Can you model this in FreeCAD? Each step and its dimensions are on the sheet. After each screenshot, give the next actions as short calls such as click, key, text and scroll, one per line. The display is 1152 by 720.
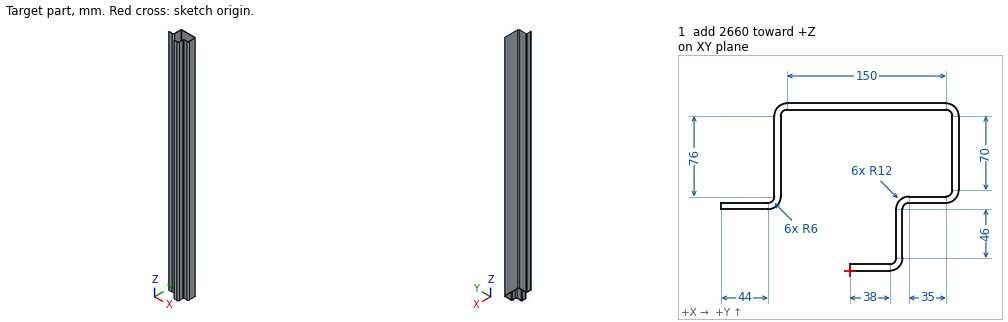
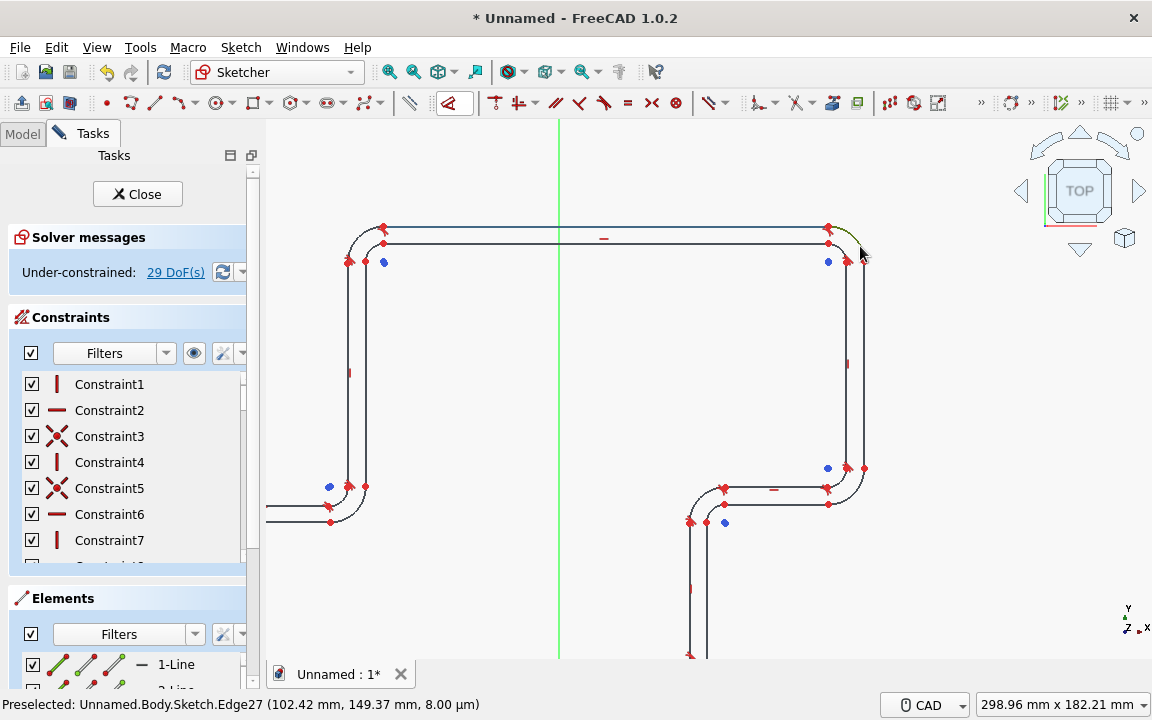
click(604, 104)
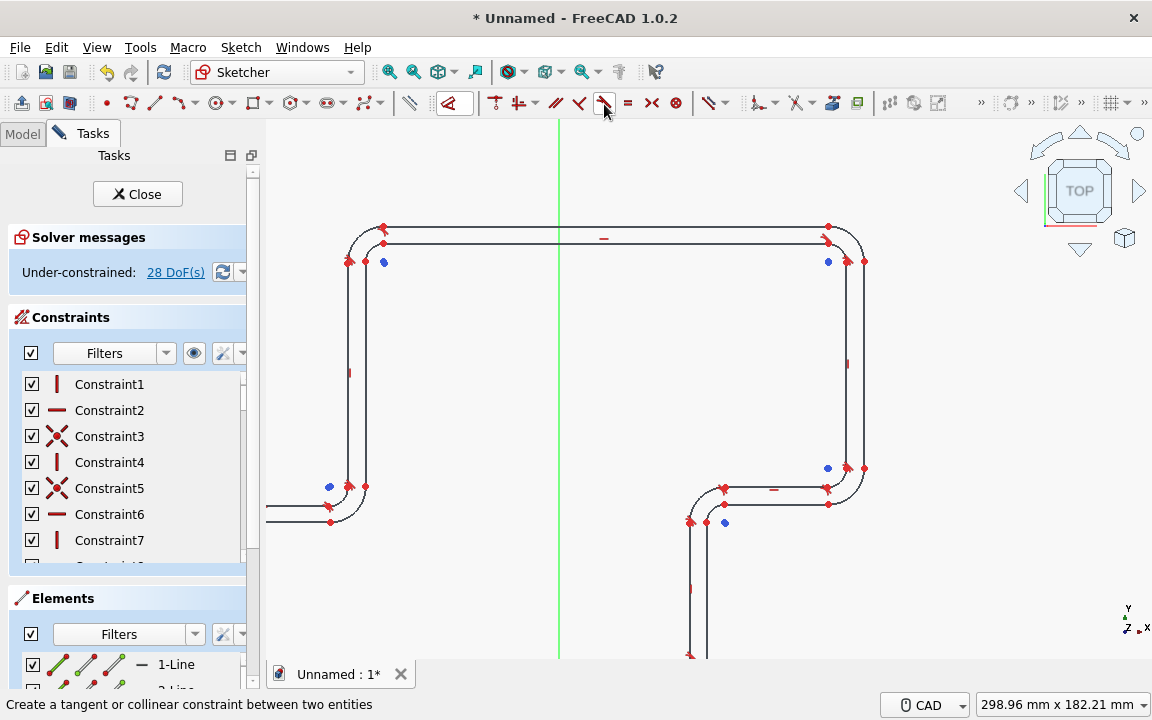
click(695, 227)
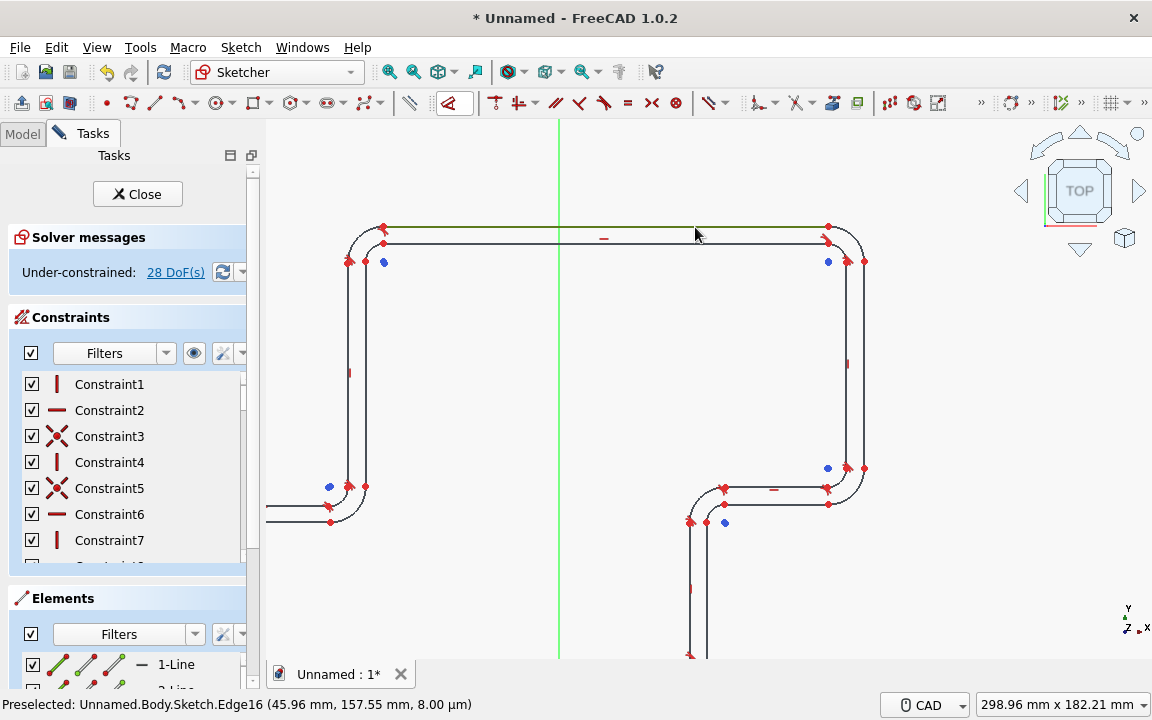
click(368, 231)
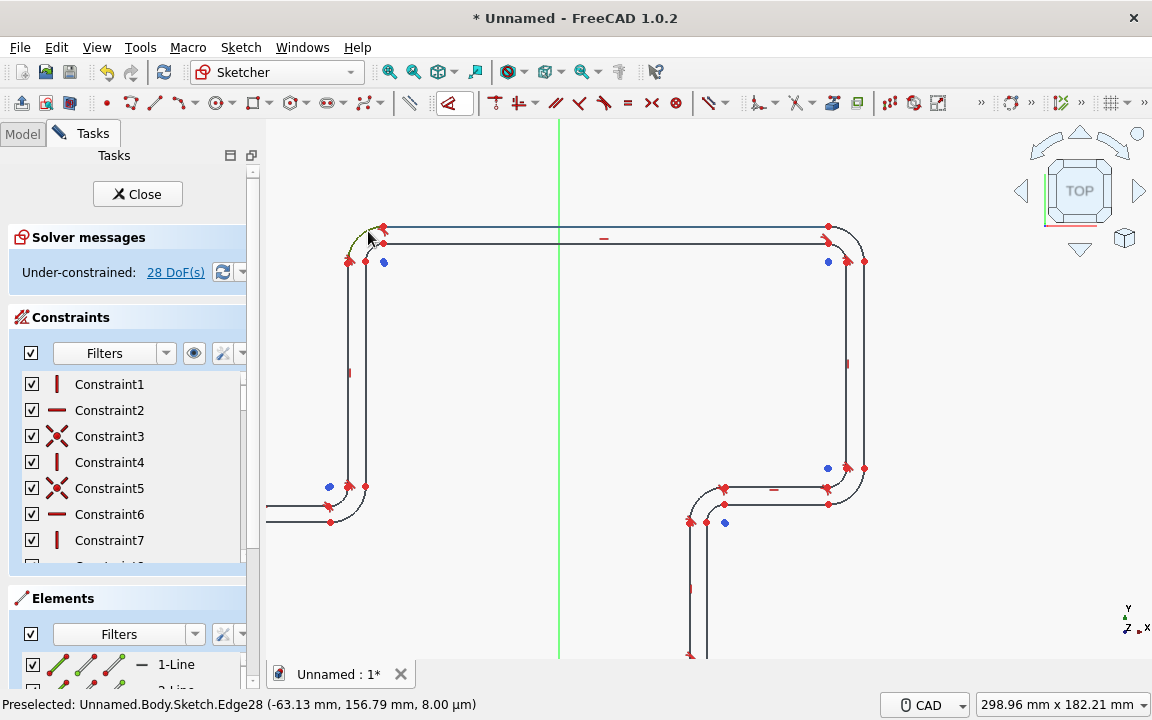
click(604, 104)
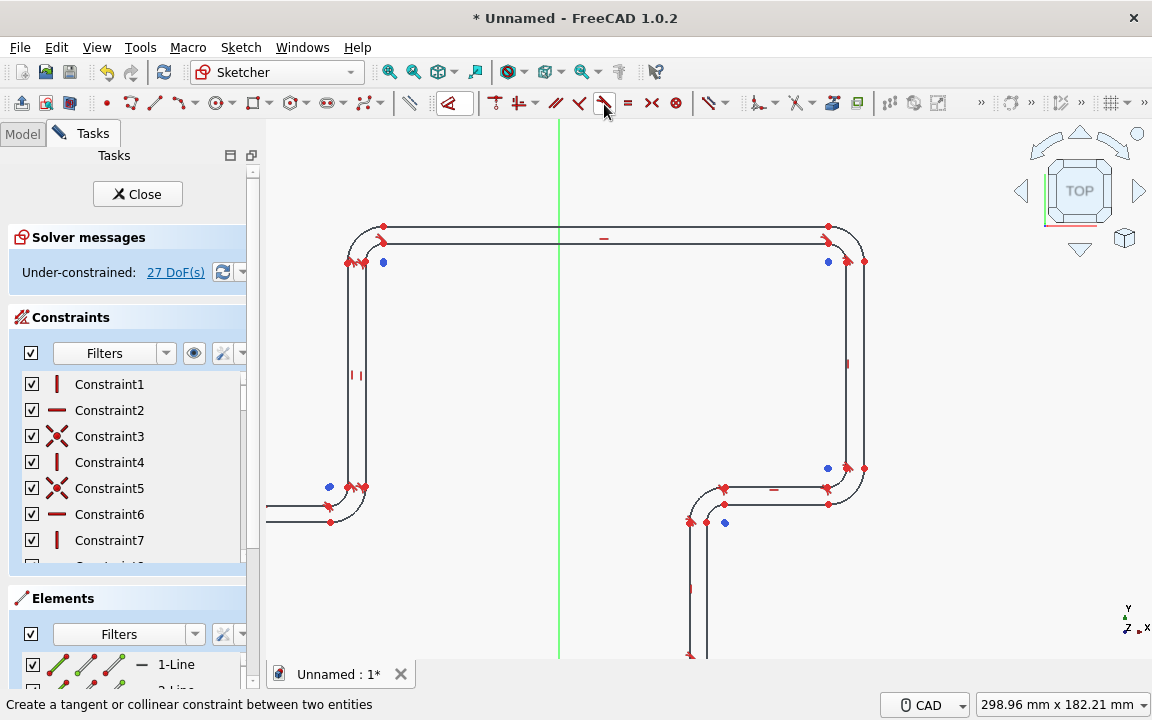
scroll(861, 246, down, 2)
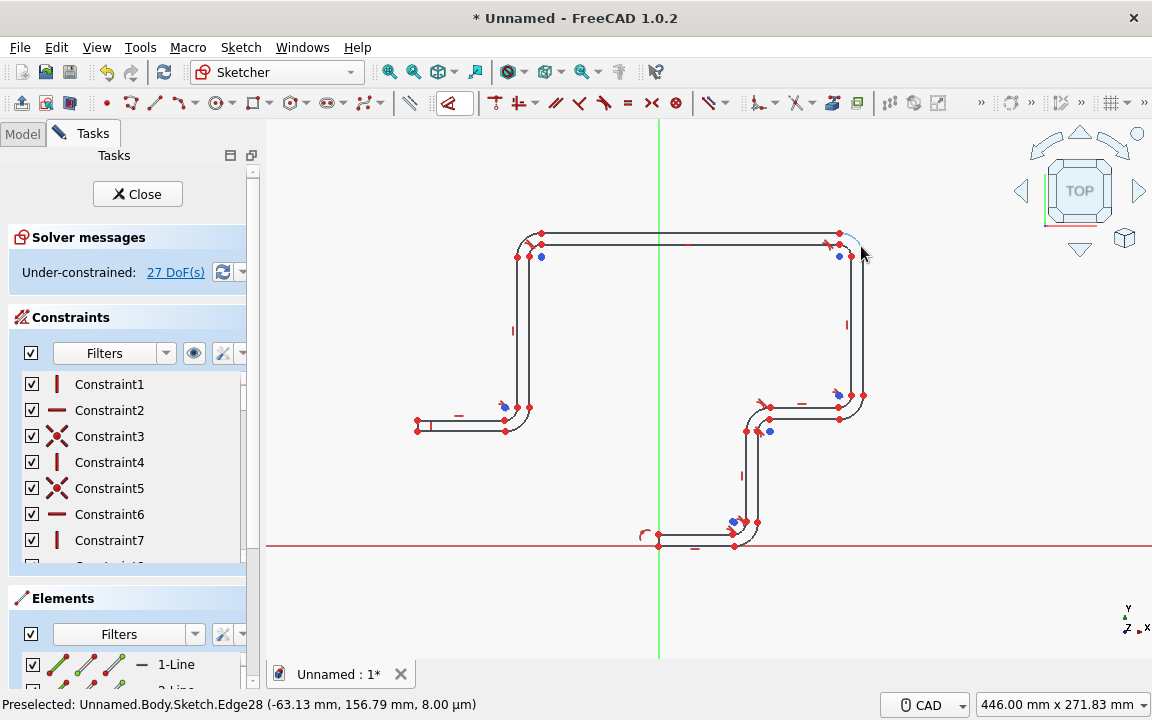
scroll(681, 546, up, 2)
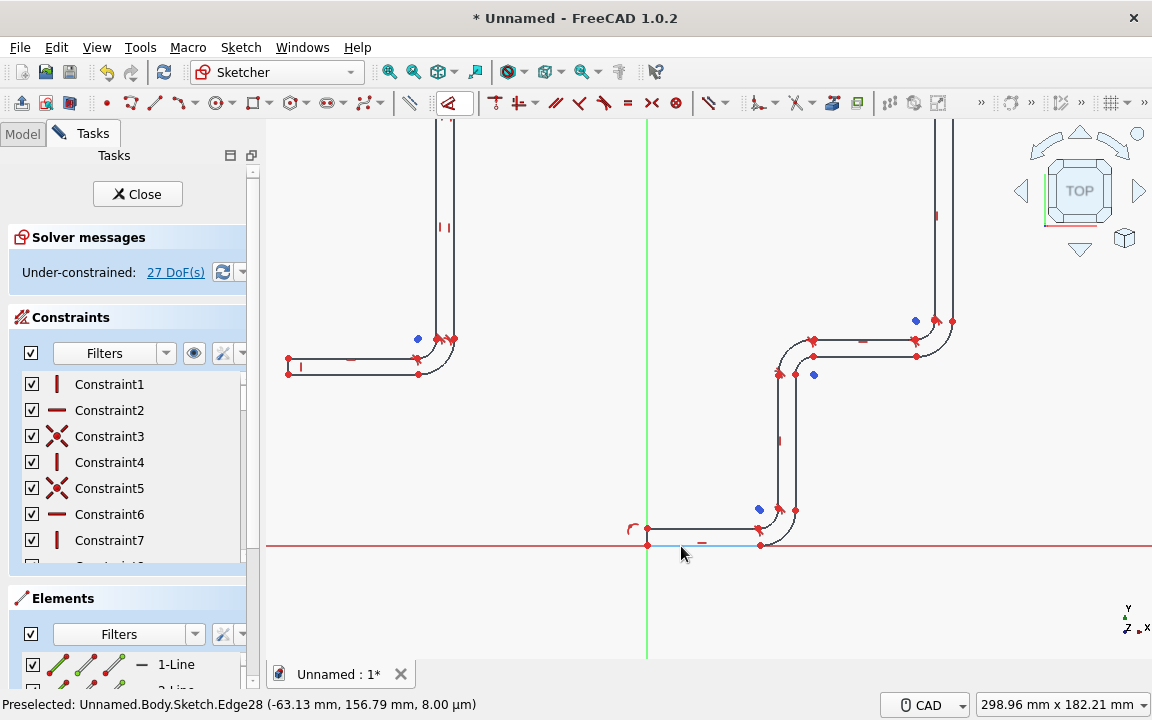
click(681, 546)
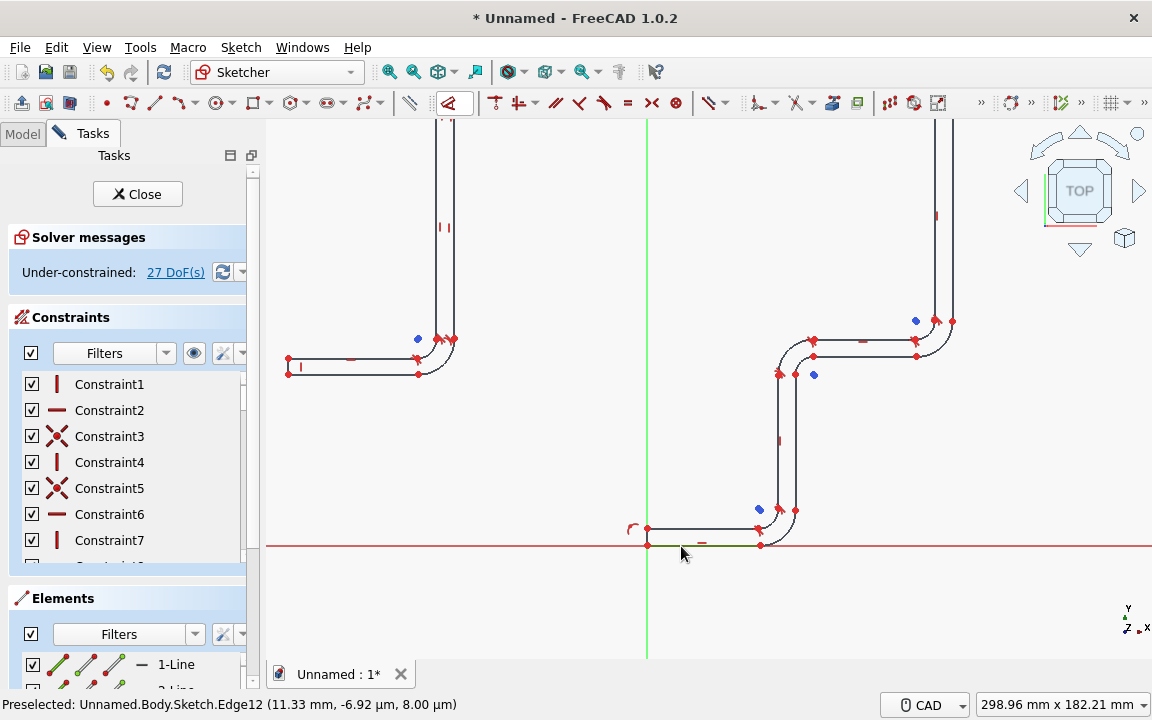
key(h)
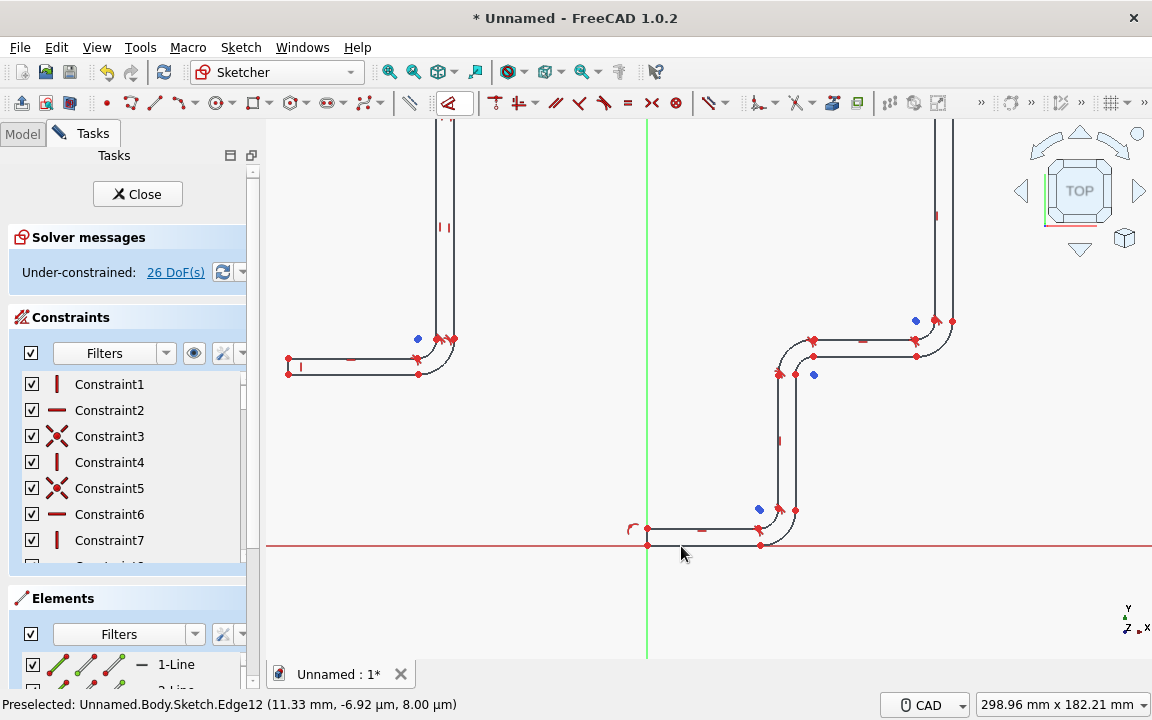
click(431, 353)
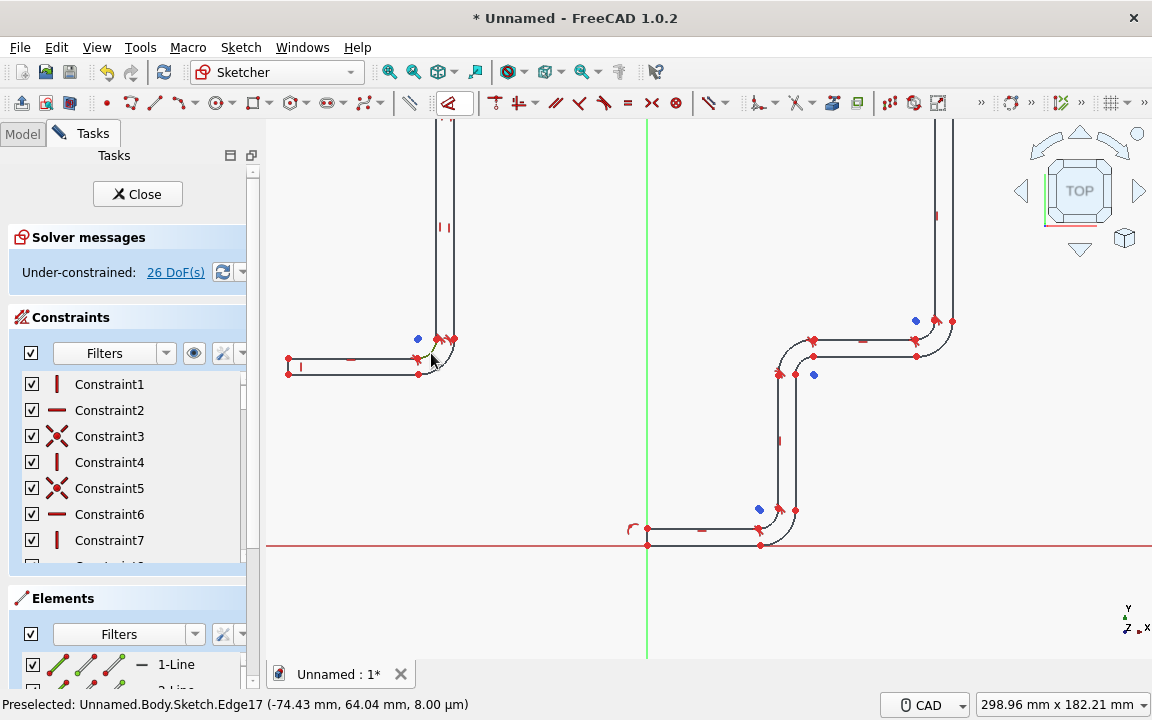
click(435, 371)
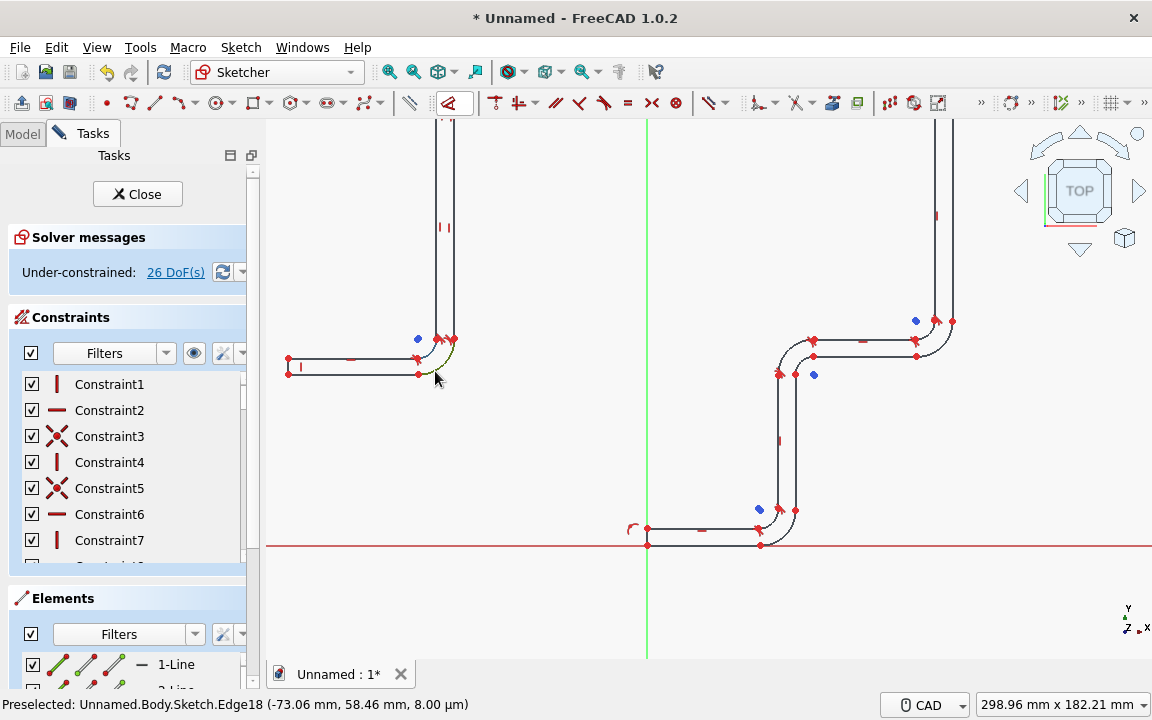
key(c)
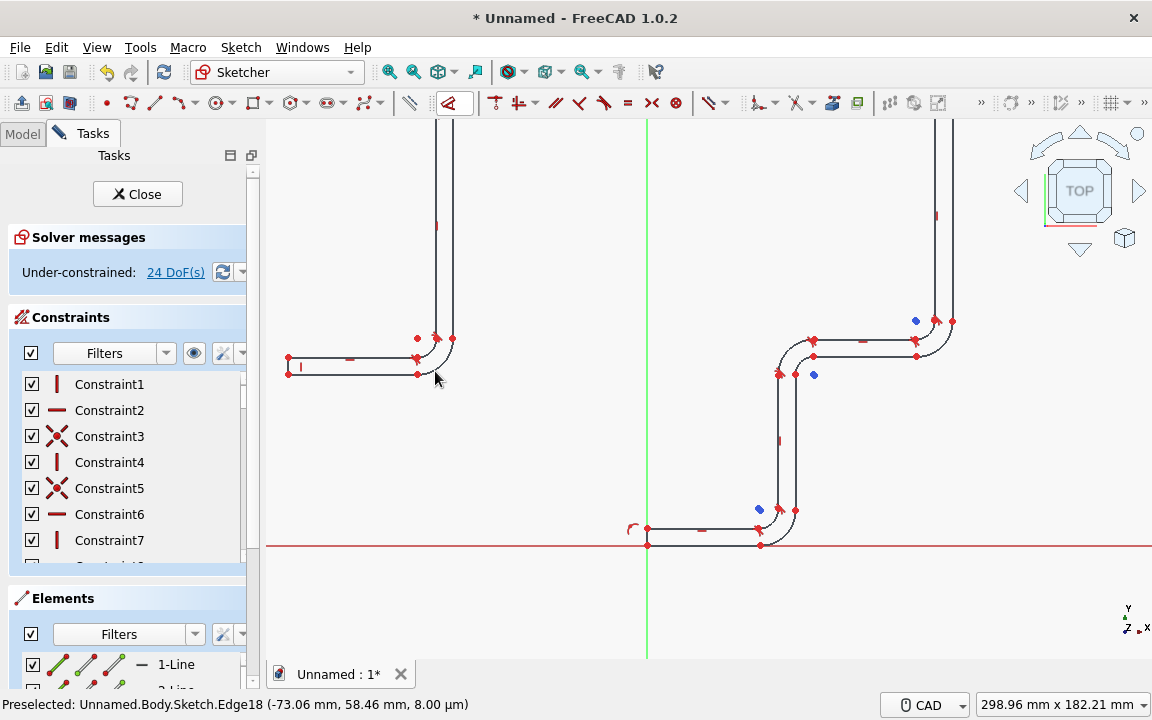
scroll(767, 527, up, 2)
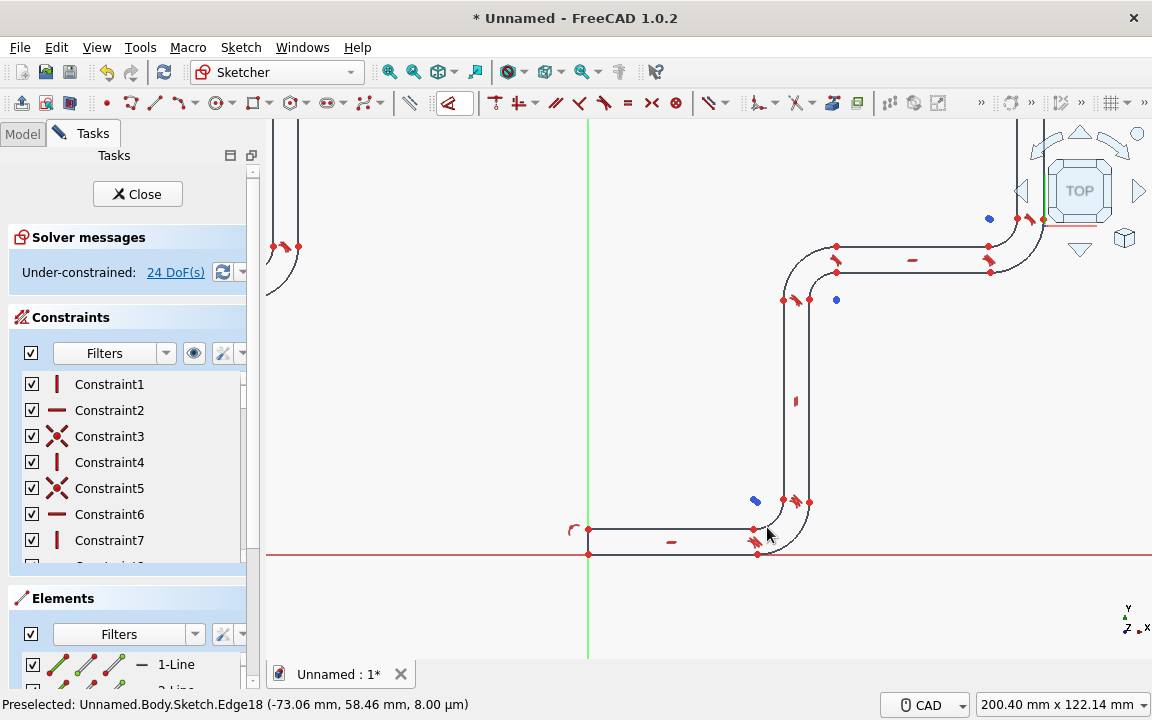
click(767, 526)